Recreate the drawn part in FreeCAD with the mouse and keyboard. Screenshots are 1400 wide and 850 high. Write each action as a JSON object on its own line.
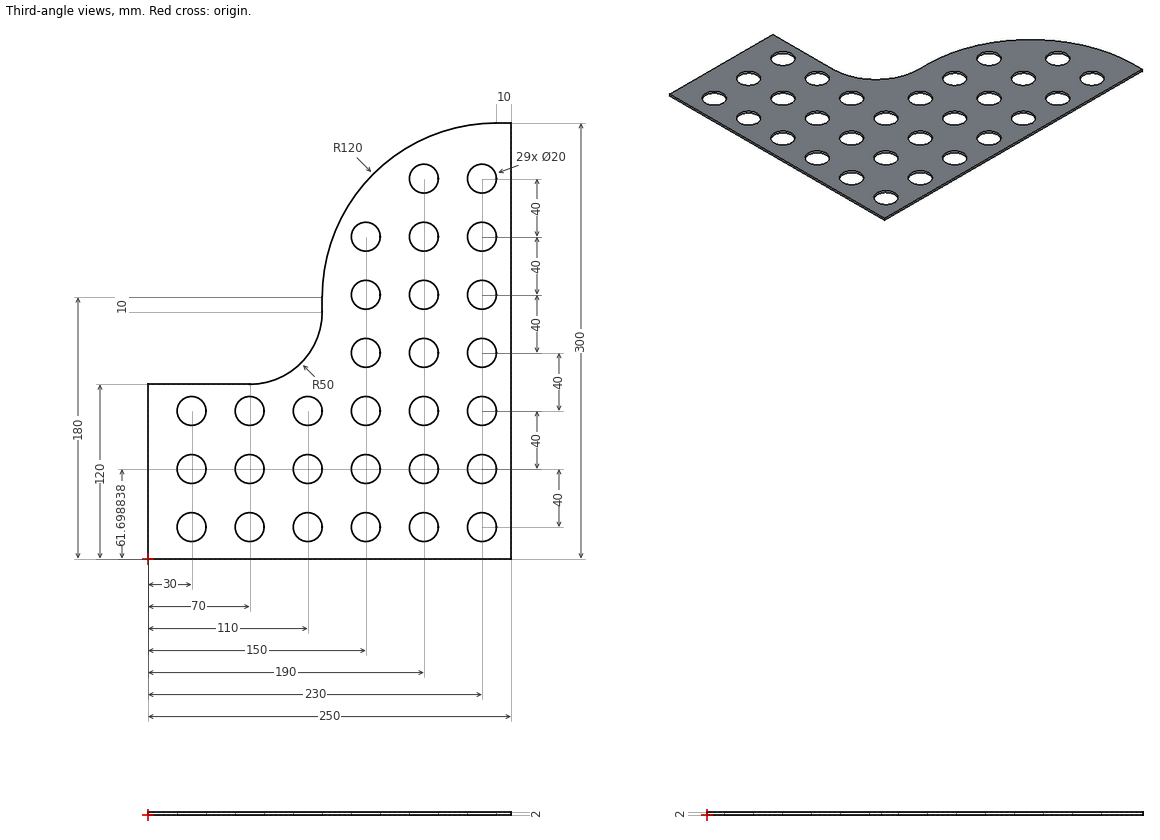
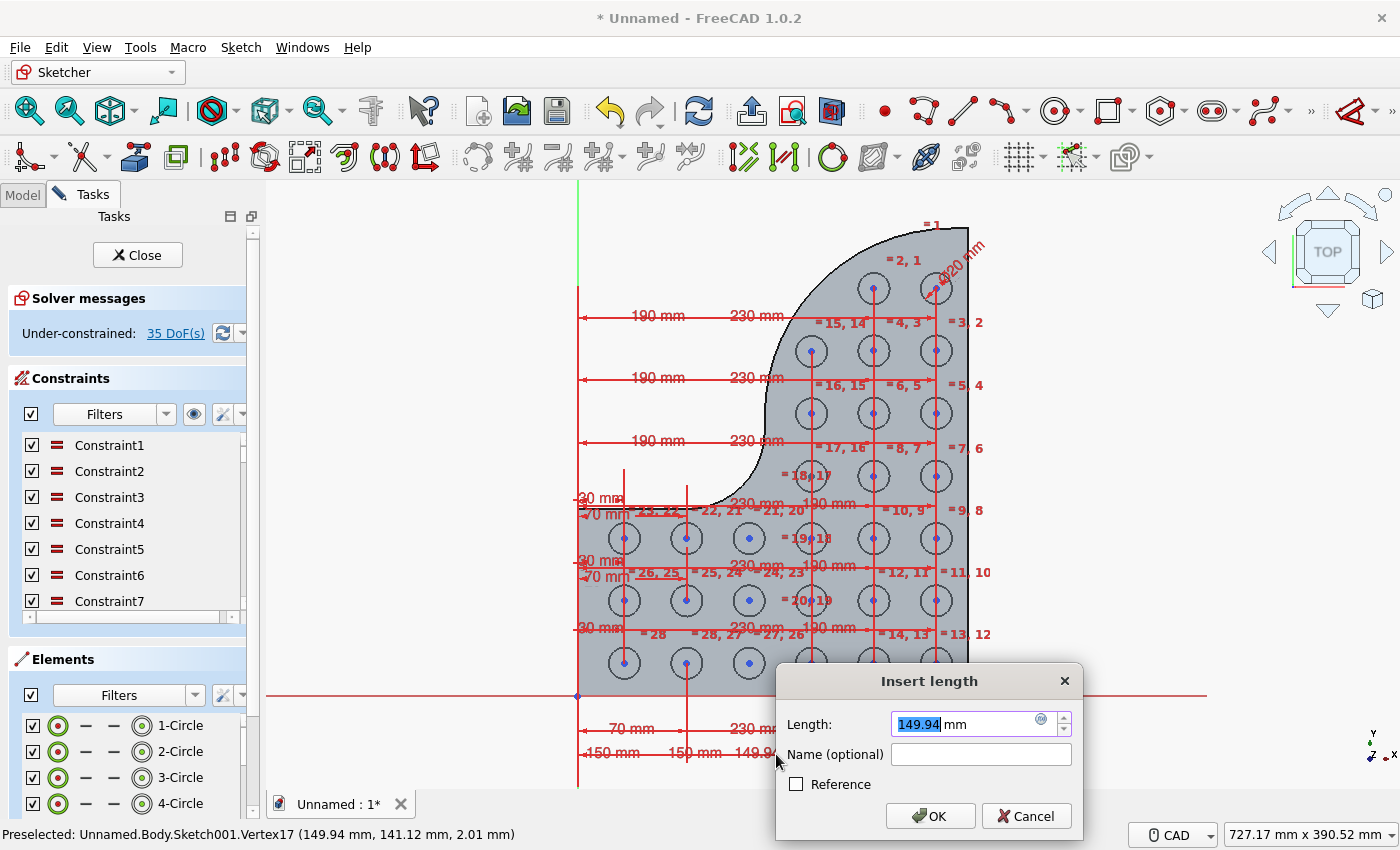
{"action": "type", "text": "150"}
{"action": "key", "text": "Return"}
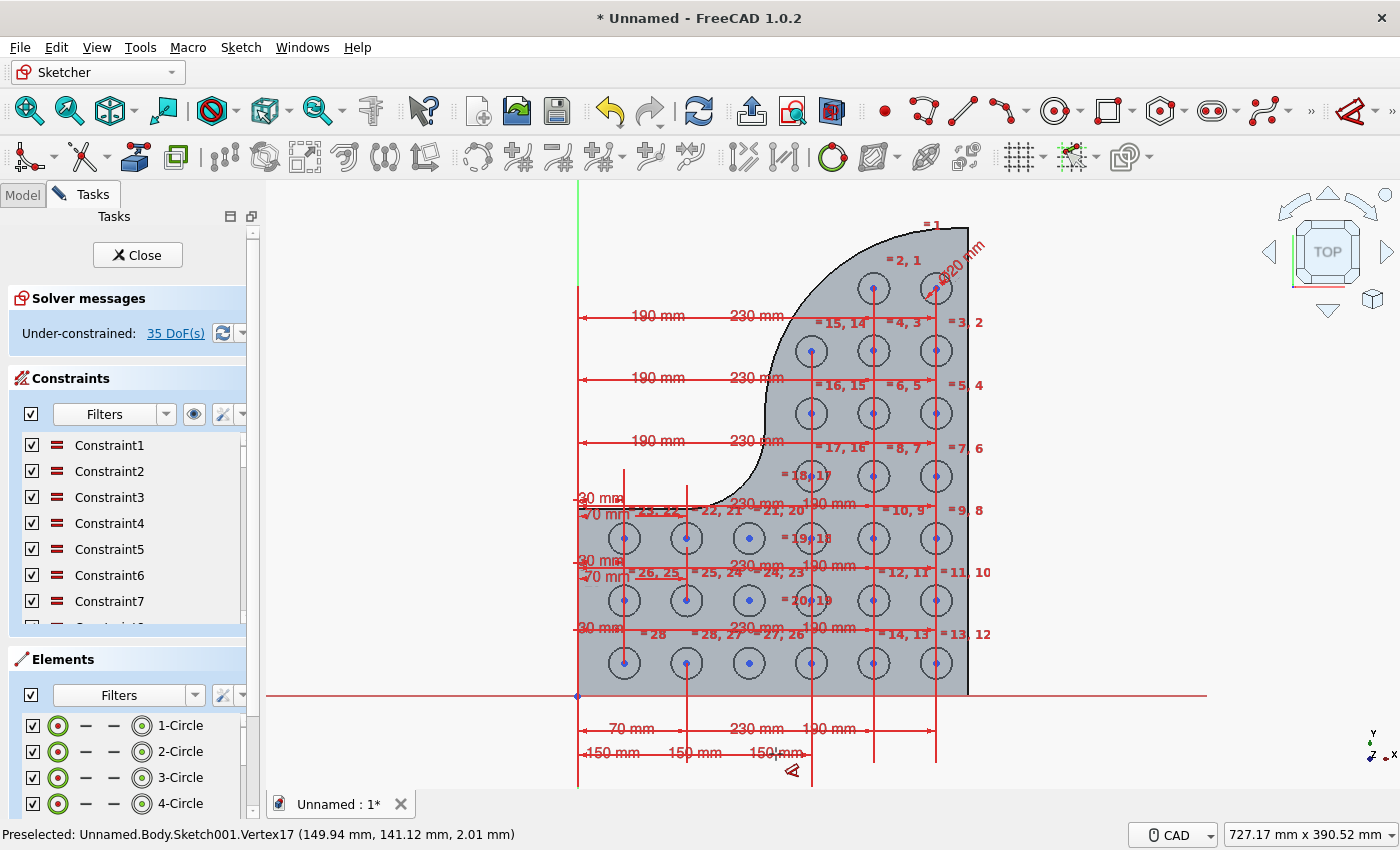
{"action": "left_click", "coordinate": [812, 539]}
{"action": "left_click", "coordinate": [695, 481]}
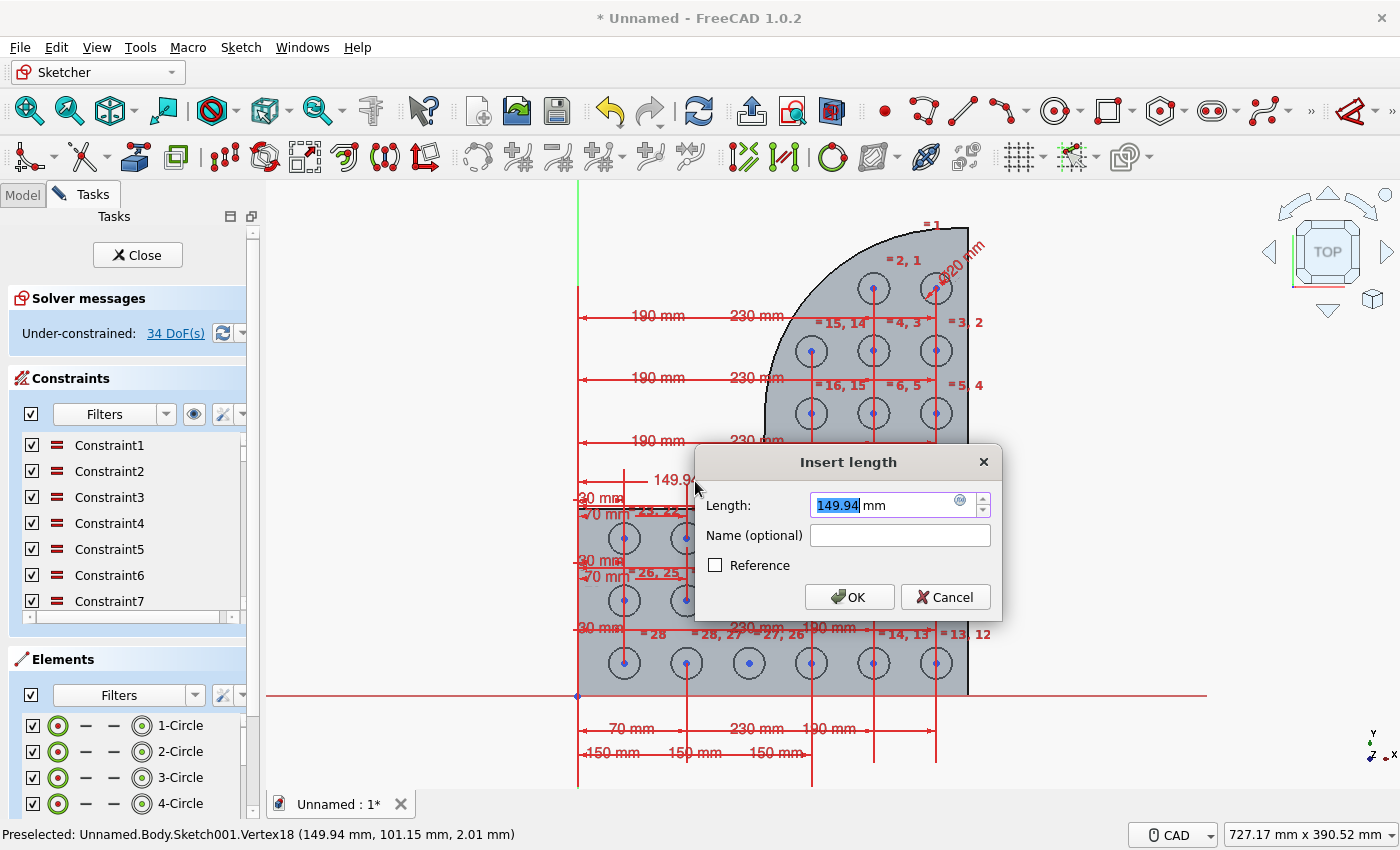
{"action": "type", "text": "150"}
{"action": "key", "text": "Return"}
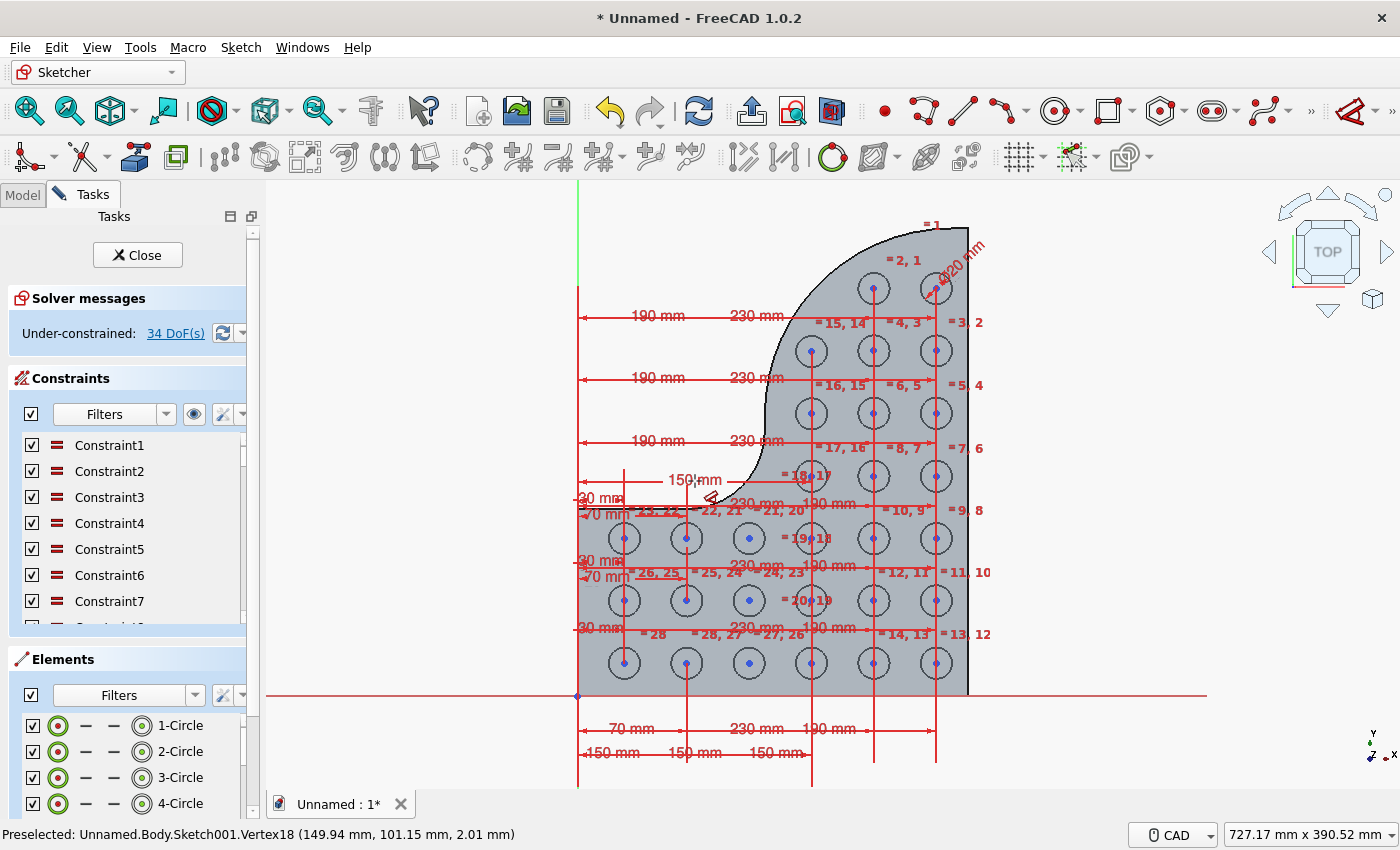
{"action": "left_click", "coordinate": [812, 601]}
{"action": "left_click", "coordinate": [613, 471]}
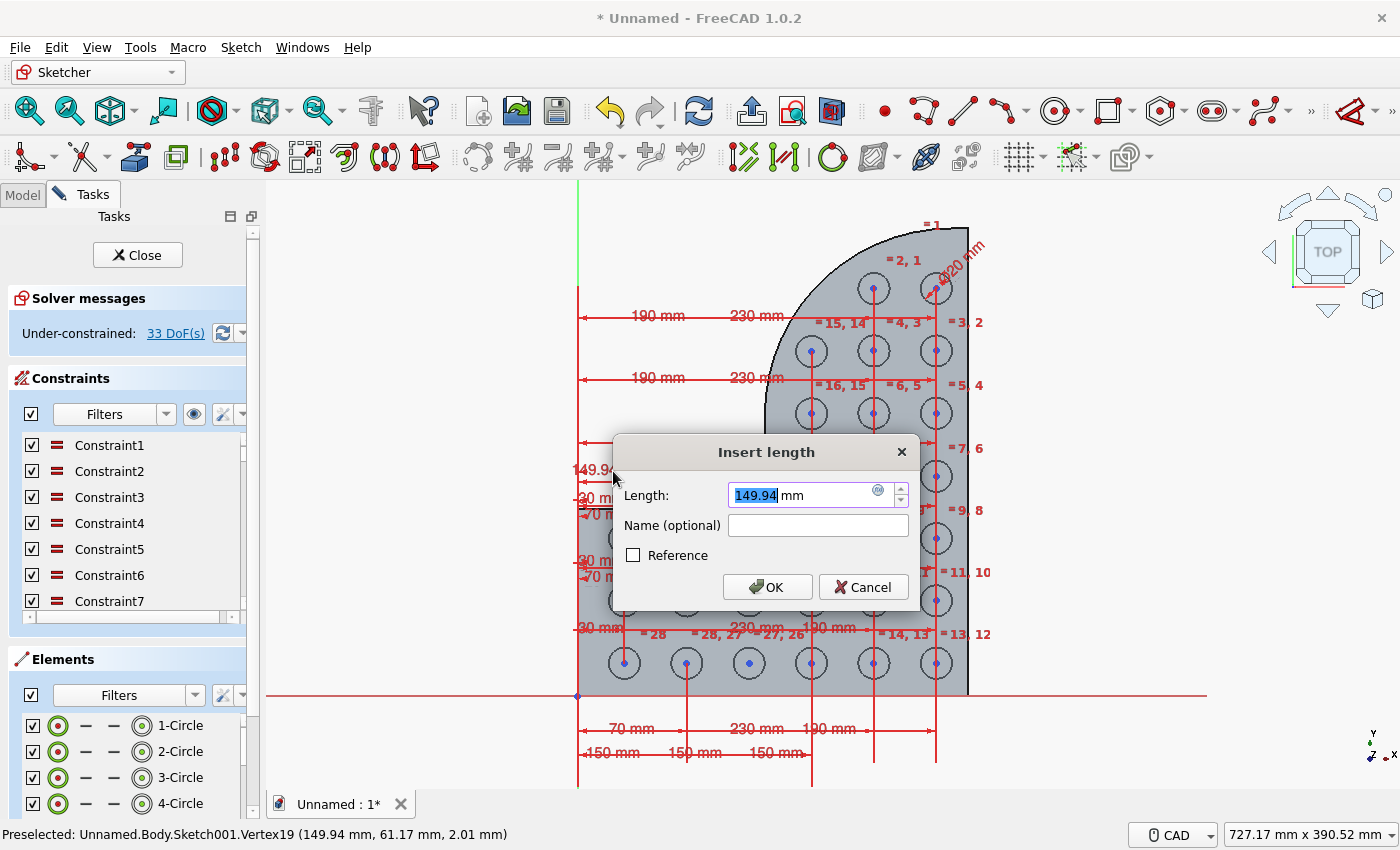
{"action": "type", "text": "150"}
{"action": "key", "text": "Return"}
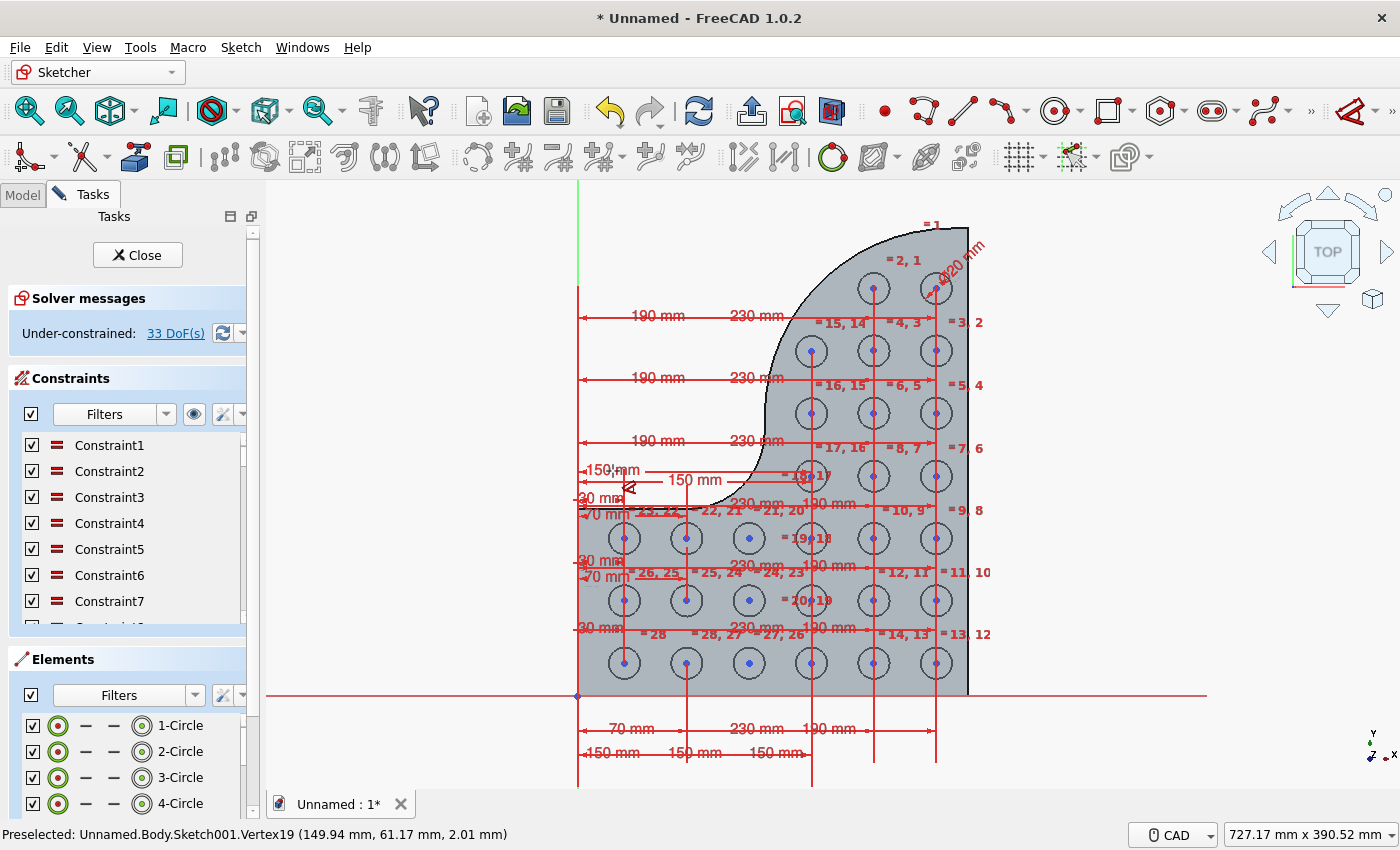
{"action": "left_click", "coordinate": [812, 663]}
{"action": "left_click", "coordinate": [776, 483]}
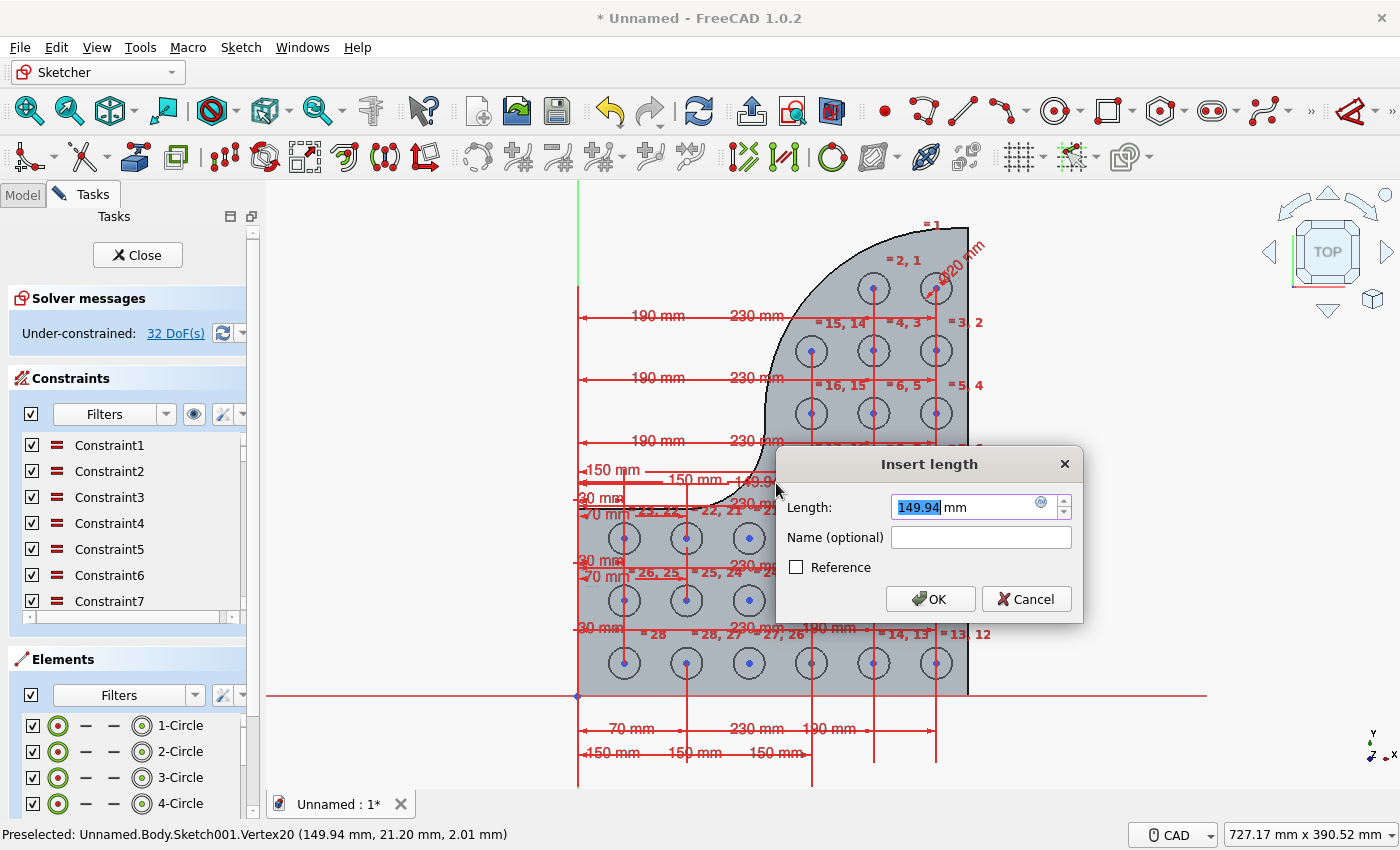
{"action": "type", "text": "150"}
{"action": "key", "text": "Return"}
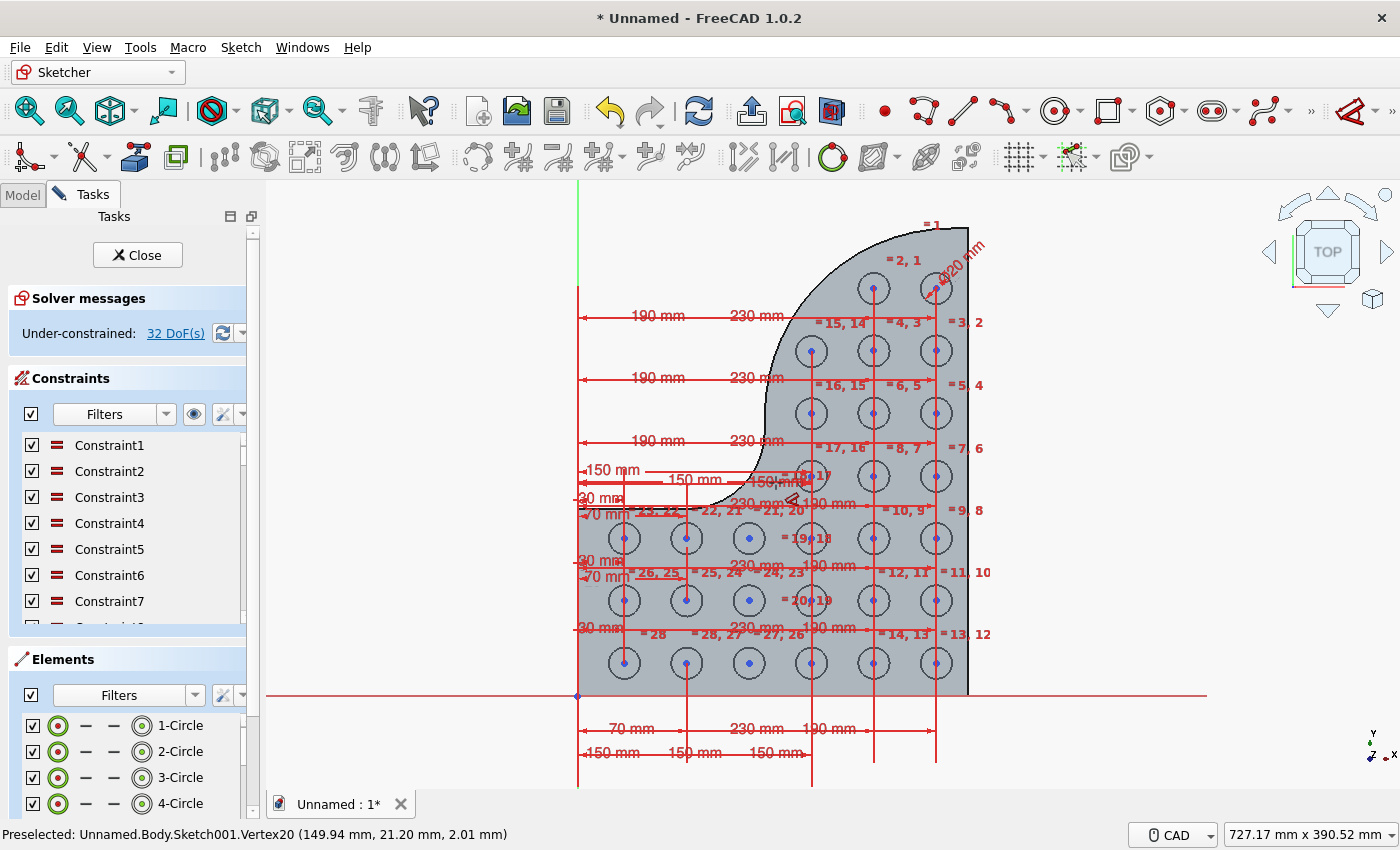
{"action": "left_click", "coordinate": [749, 539]}
{"action": "left_click", "coordinate": [663, 409]}